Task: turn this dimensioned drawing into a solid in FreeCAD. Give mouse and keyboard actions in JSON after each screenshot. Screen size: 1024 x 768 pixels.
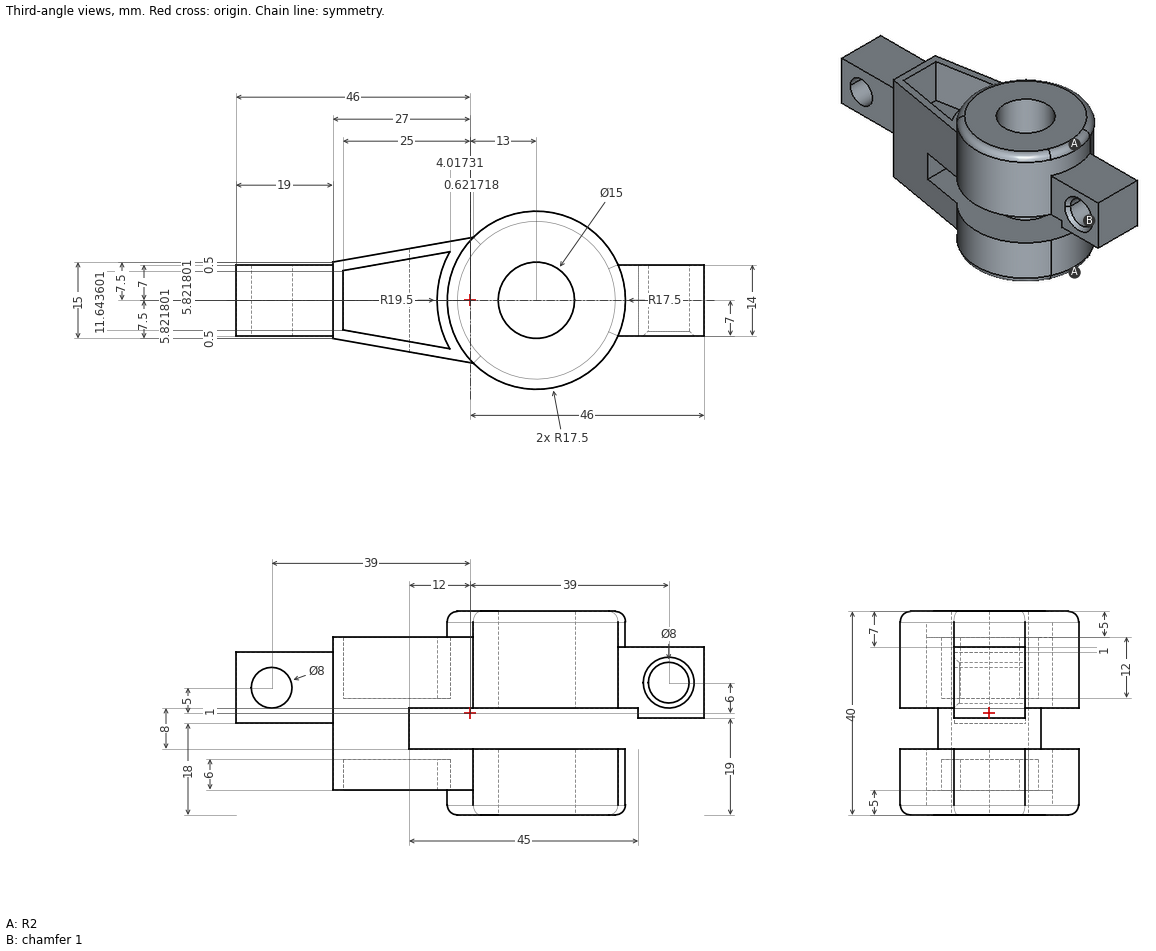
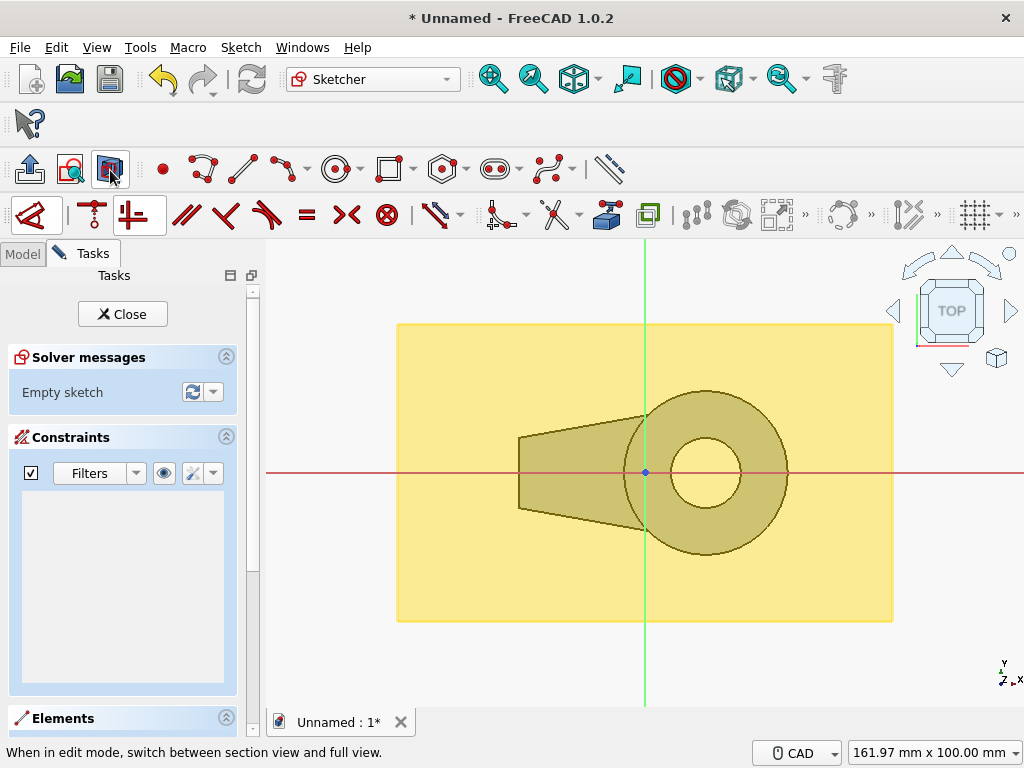
{"action": "scroll", "coordinate": [591, 473], "scroll_direction": "up", "scroll_amount": 6}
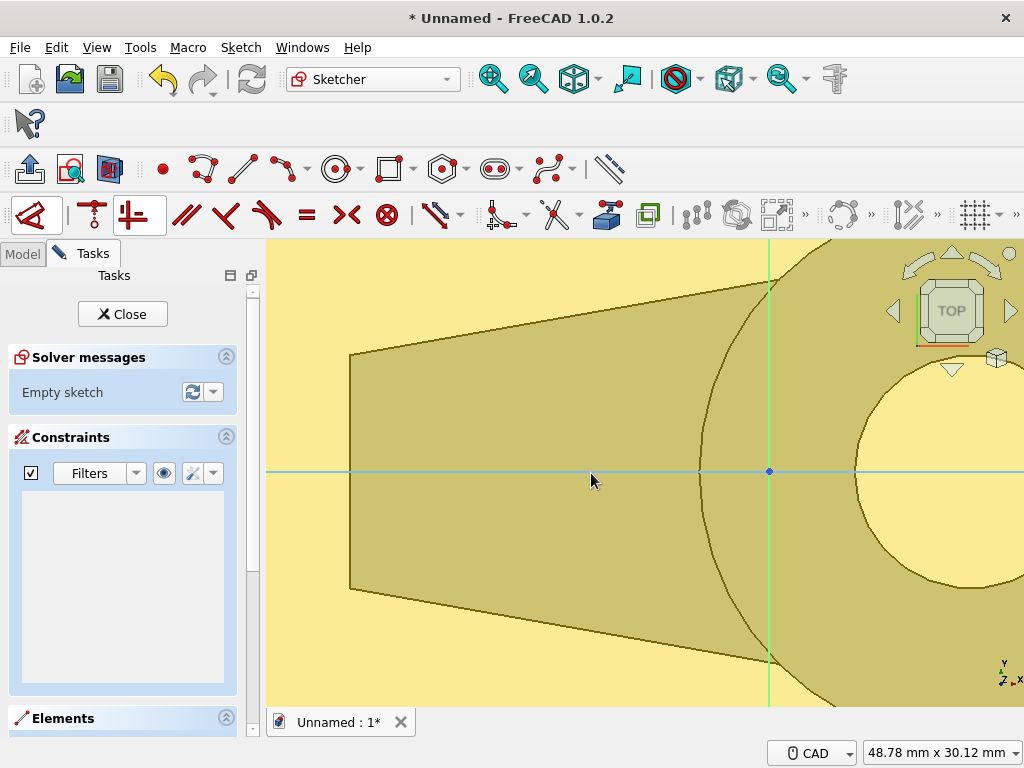
{"action": "left_click", "coordinate": [204, 170]}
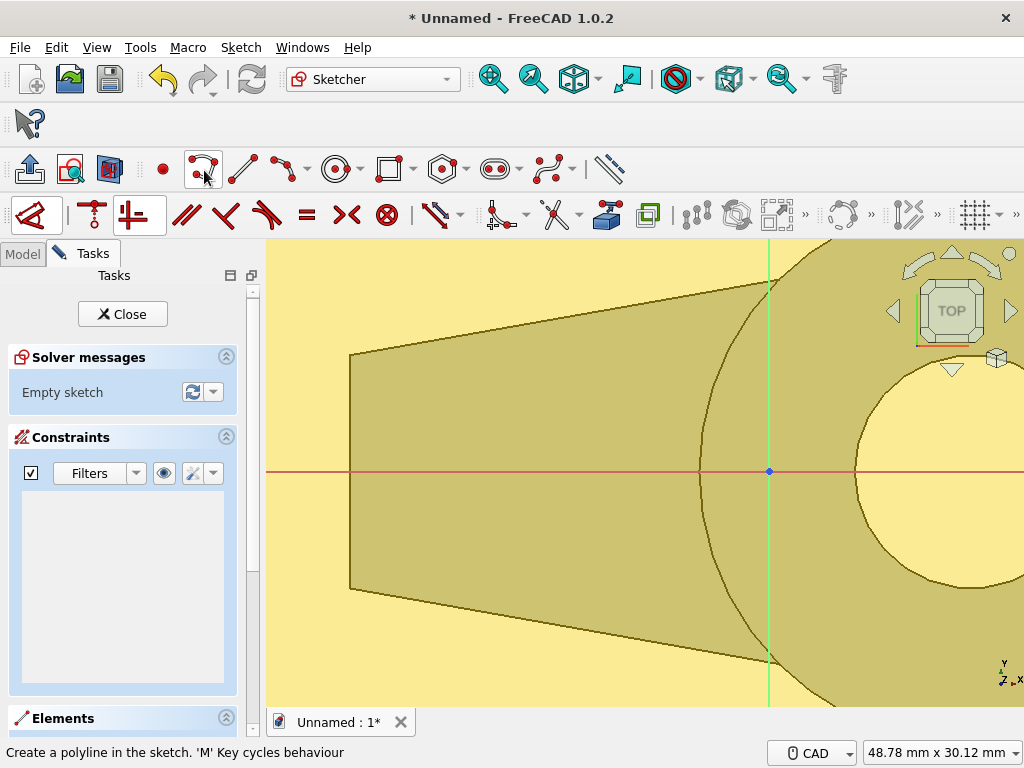
{"action": "left_click", "coordinate": [707, 620]}
{"action": "left_click", "coordinate": [381, 562]}
{"action": "left_click", "coordinate": [381, 381]}
{"action": "left_click", "coordinate": [707, 324]}
{"action": "right_click", "coordinate": [707, 324]}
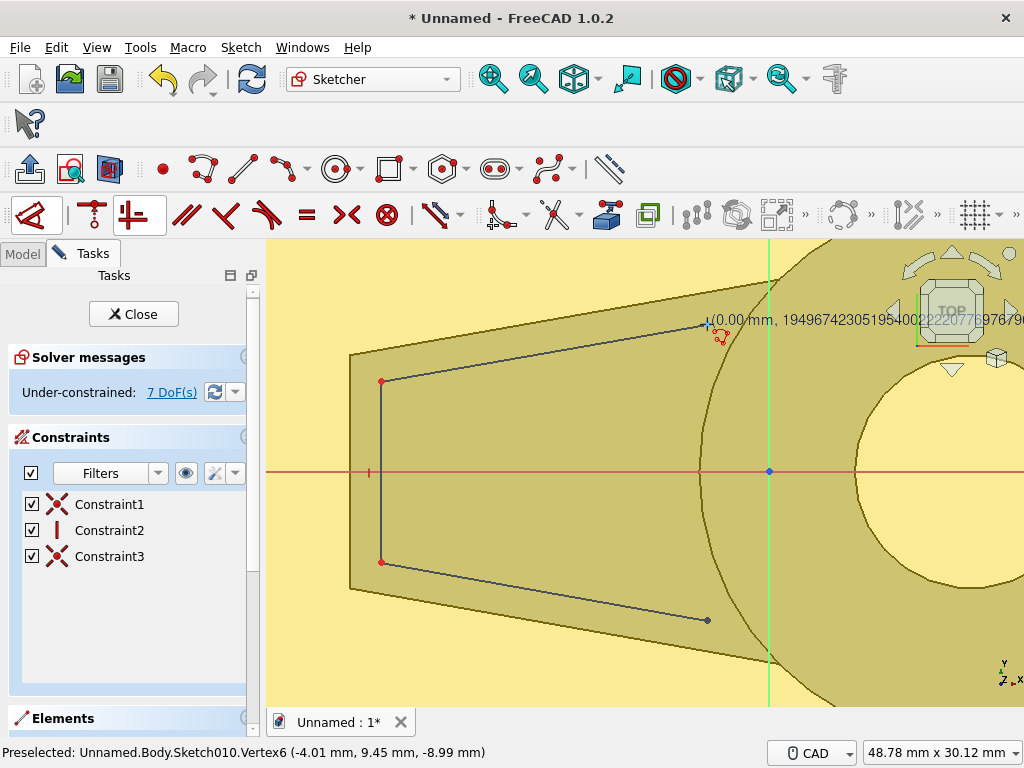
{"action": "left_click", "coordinate": [284, 170]}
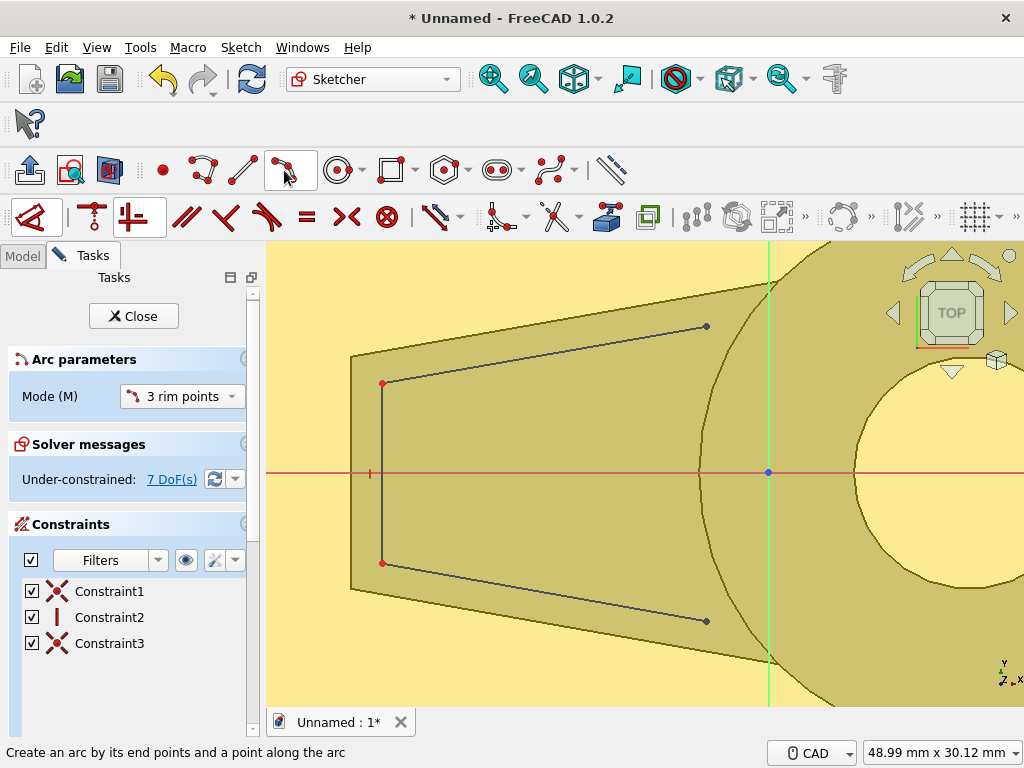
{"action": "left_click", "coordinate": [707, 327]}
{"action": "left_click", "coordinate": [707, 621]}
{"action": "left_click", "coordinate": [670, 442]}
{"action": "key", "text": "Escape"}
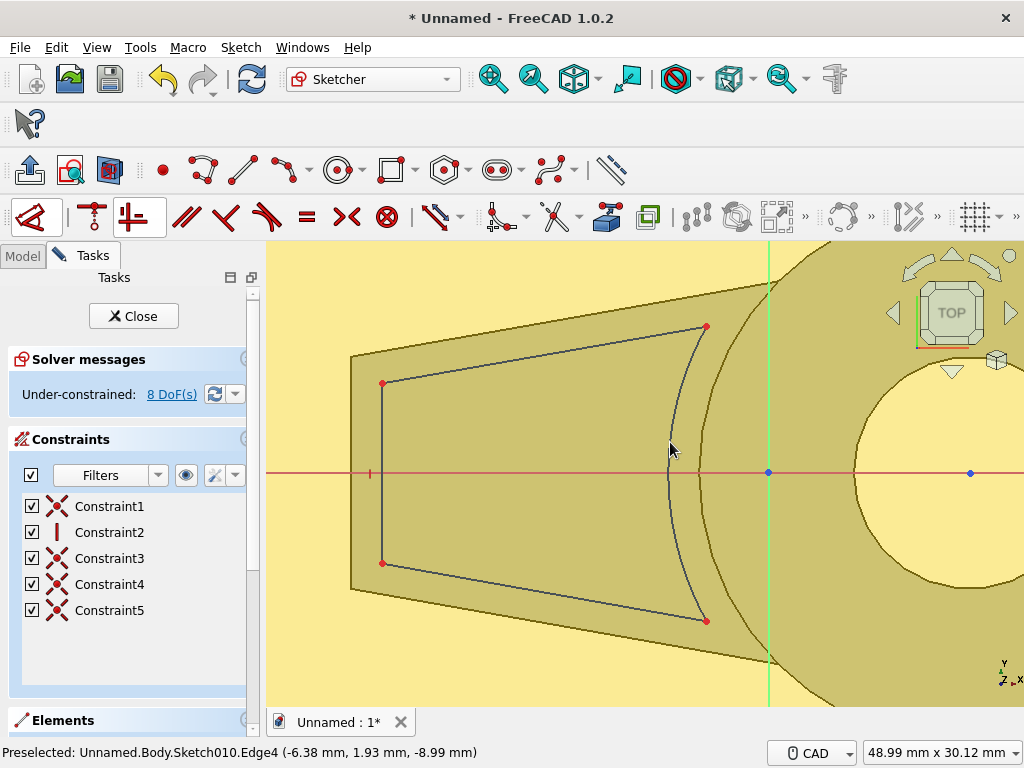
{"action": "scroll", "coordinate": [373, 476], "scroll_direction": "down", "scroll_amount": 2}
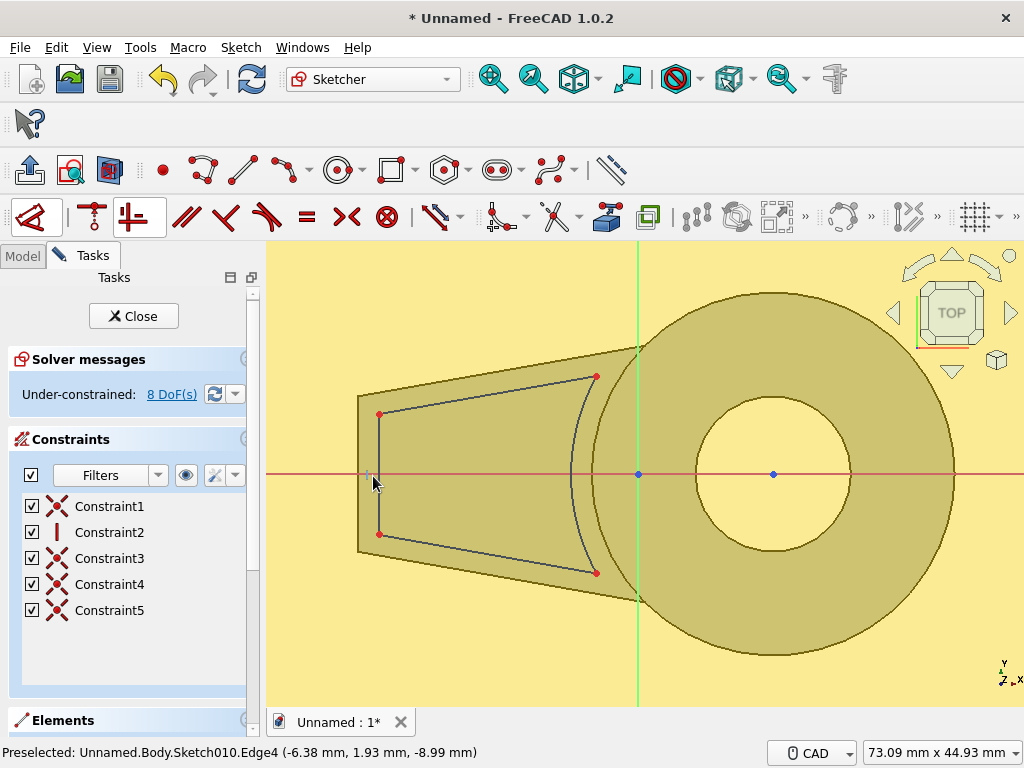
{"action": "left_click", "coordinate": [774, 475]}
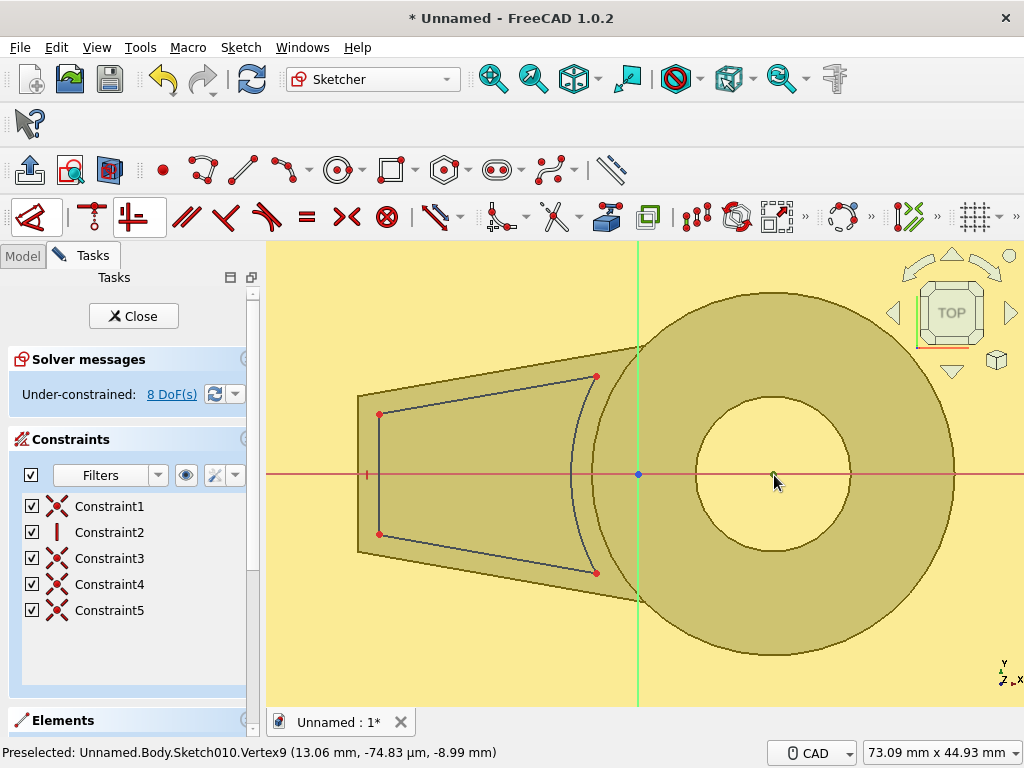
{"action": "left_click", "coordinate": [334, 474]}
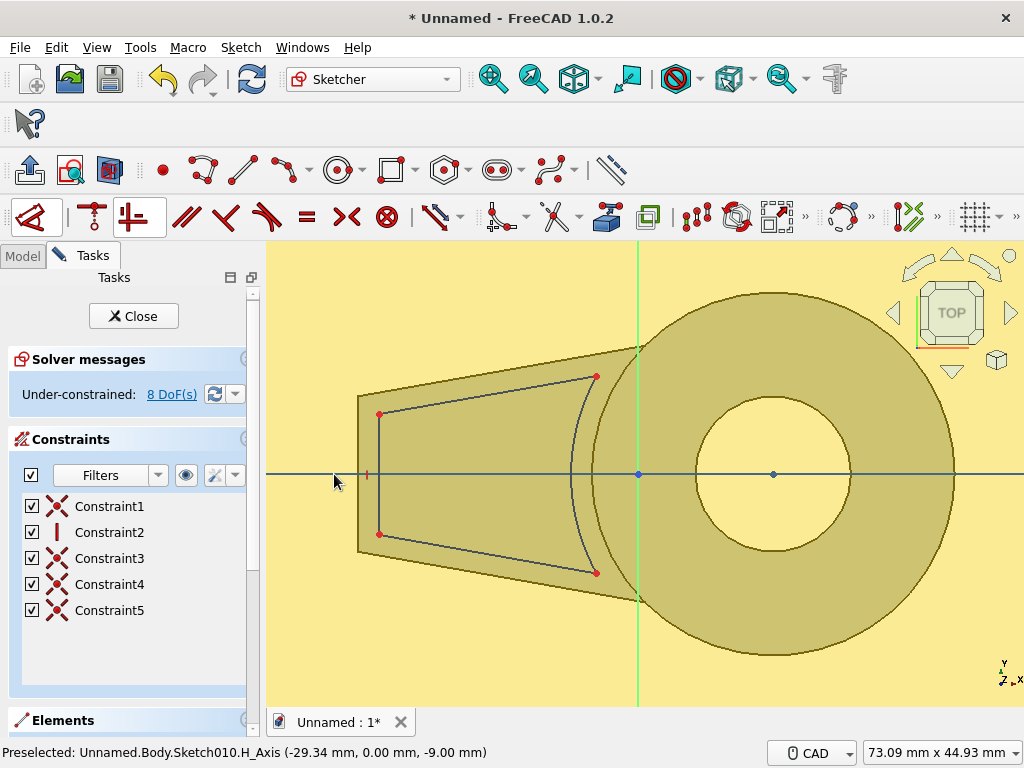
{"action": "left_click", "coordinate": [92, 218]}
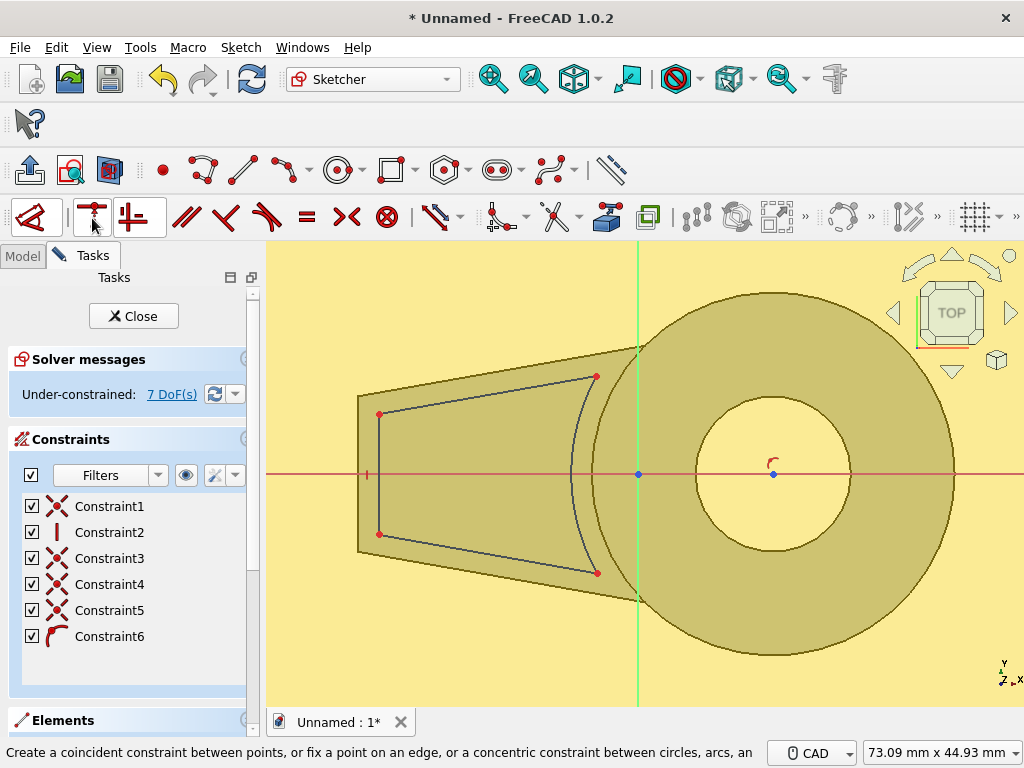
{"action": "left_click", "coordinate": [575, 434]}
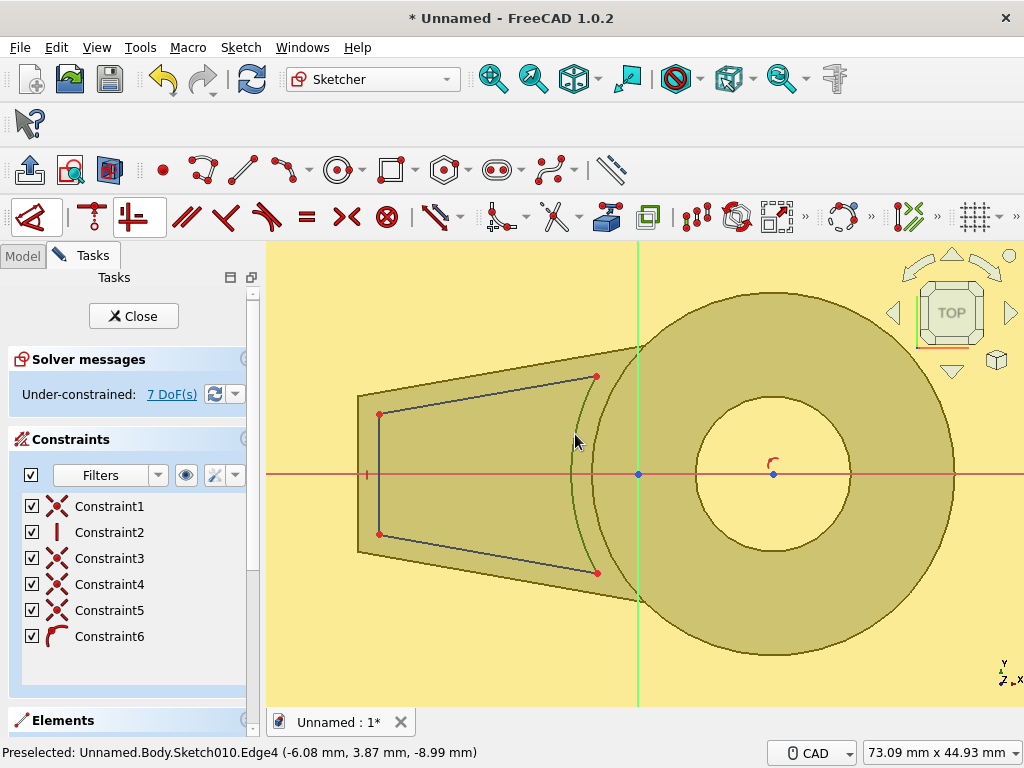
{"action": "left_click", "coordinate": [56, 218]}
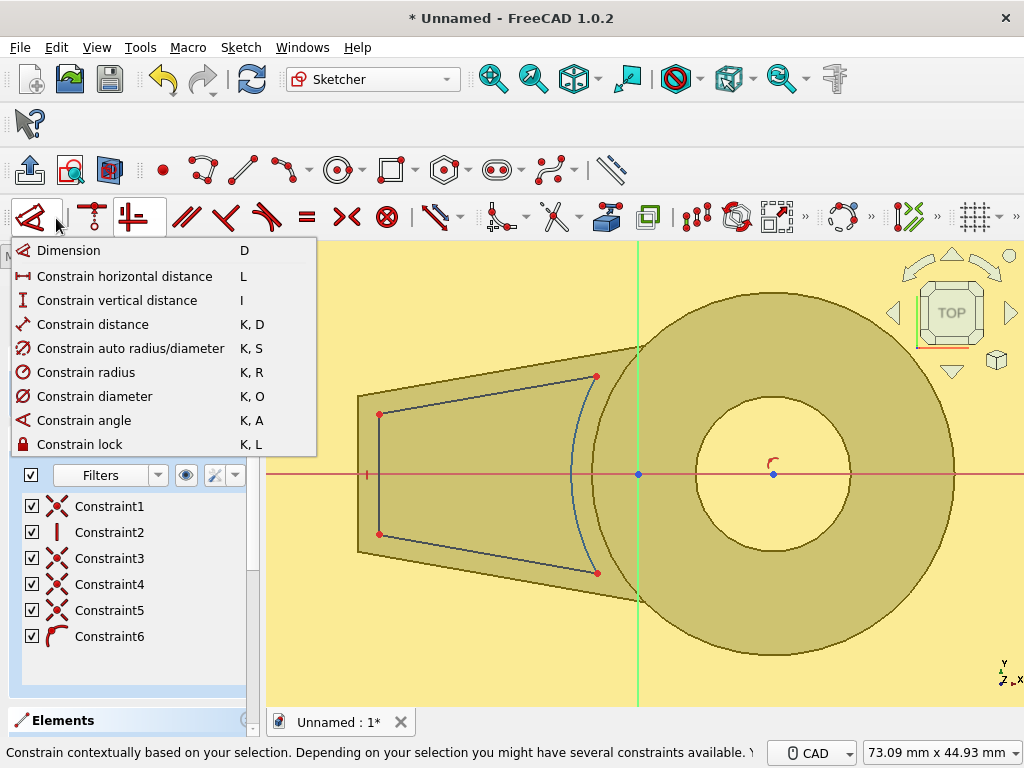
{"action": "left_click", "coordinate": [164, 372]}